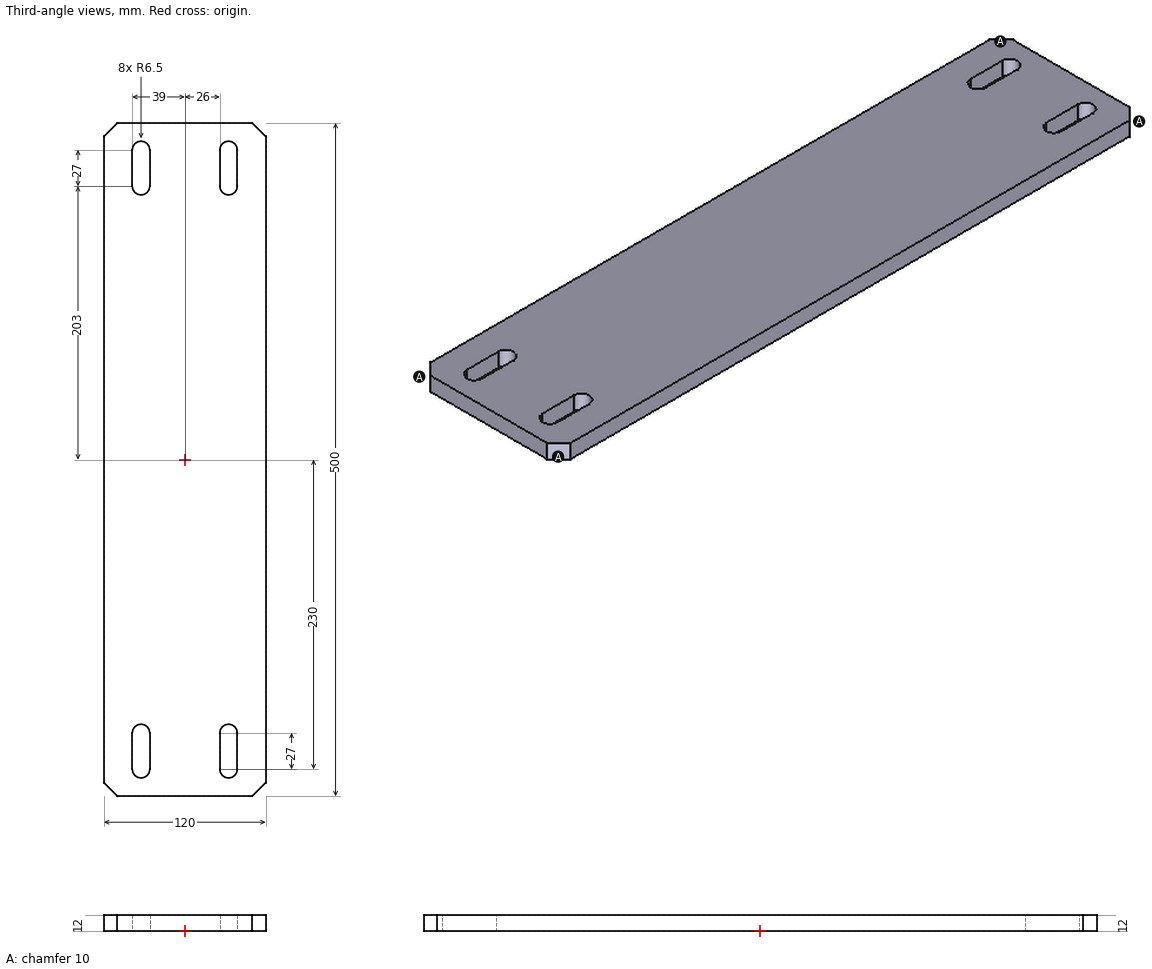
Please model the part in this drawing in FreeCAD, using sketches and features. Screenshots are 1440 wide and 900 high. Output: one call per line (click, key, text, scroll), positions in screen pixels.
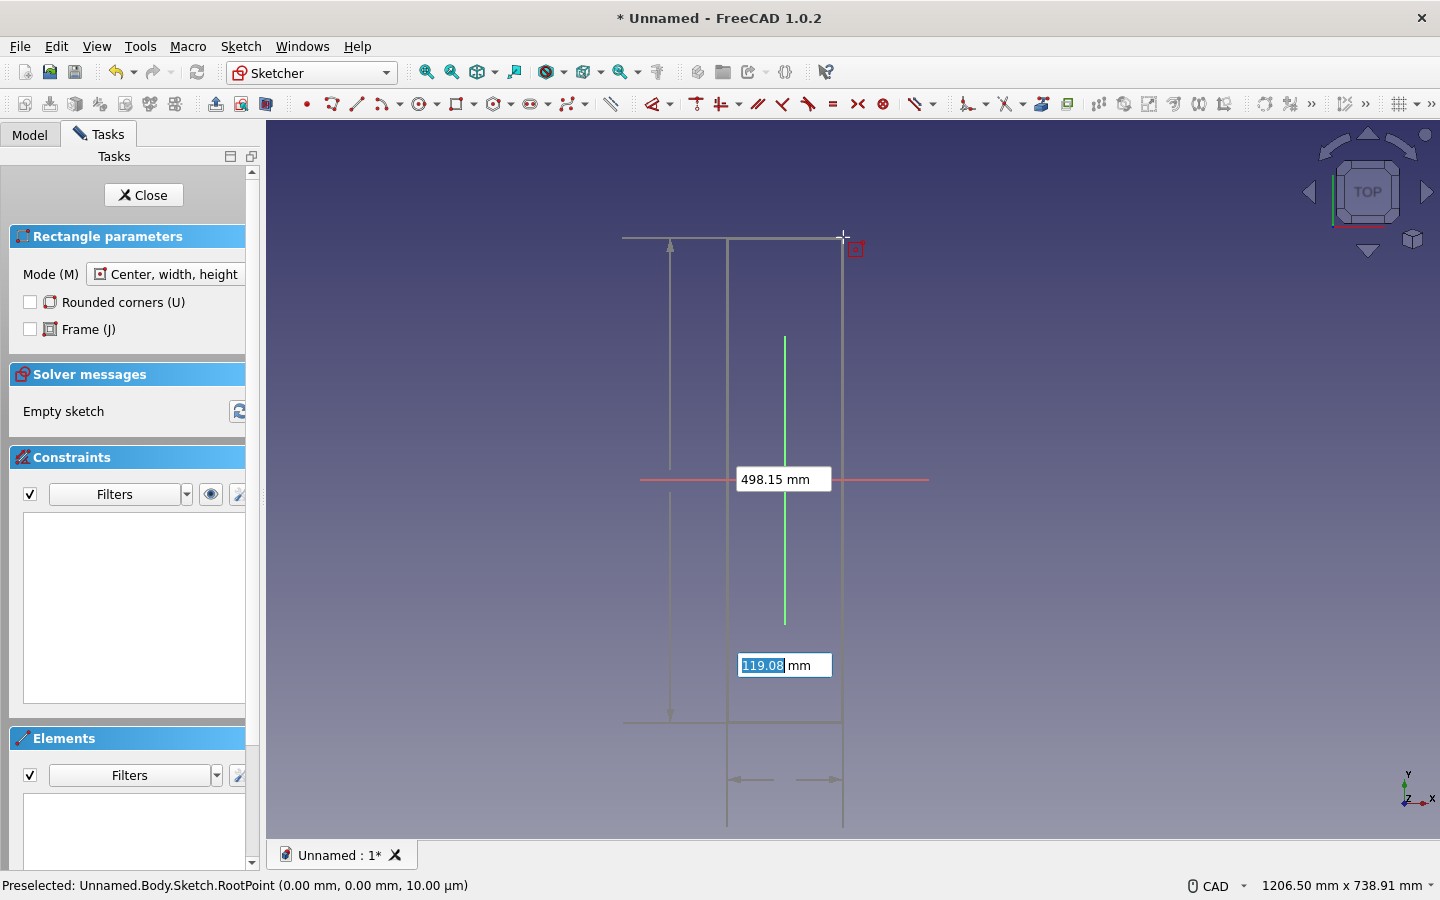
text(120)
key(Tab)
text(500)
key(Return)
key(Escape)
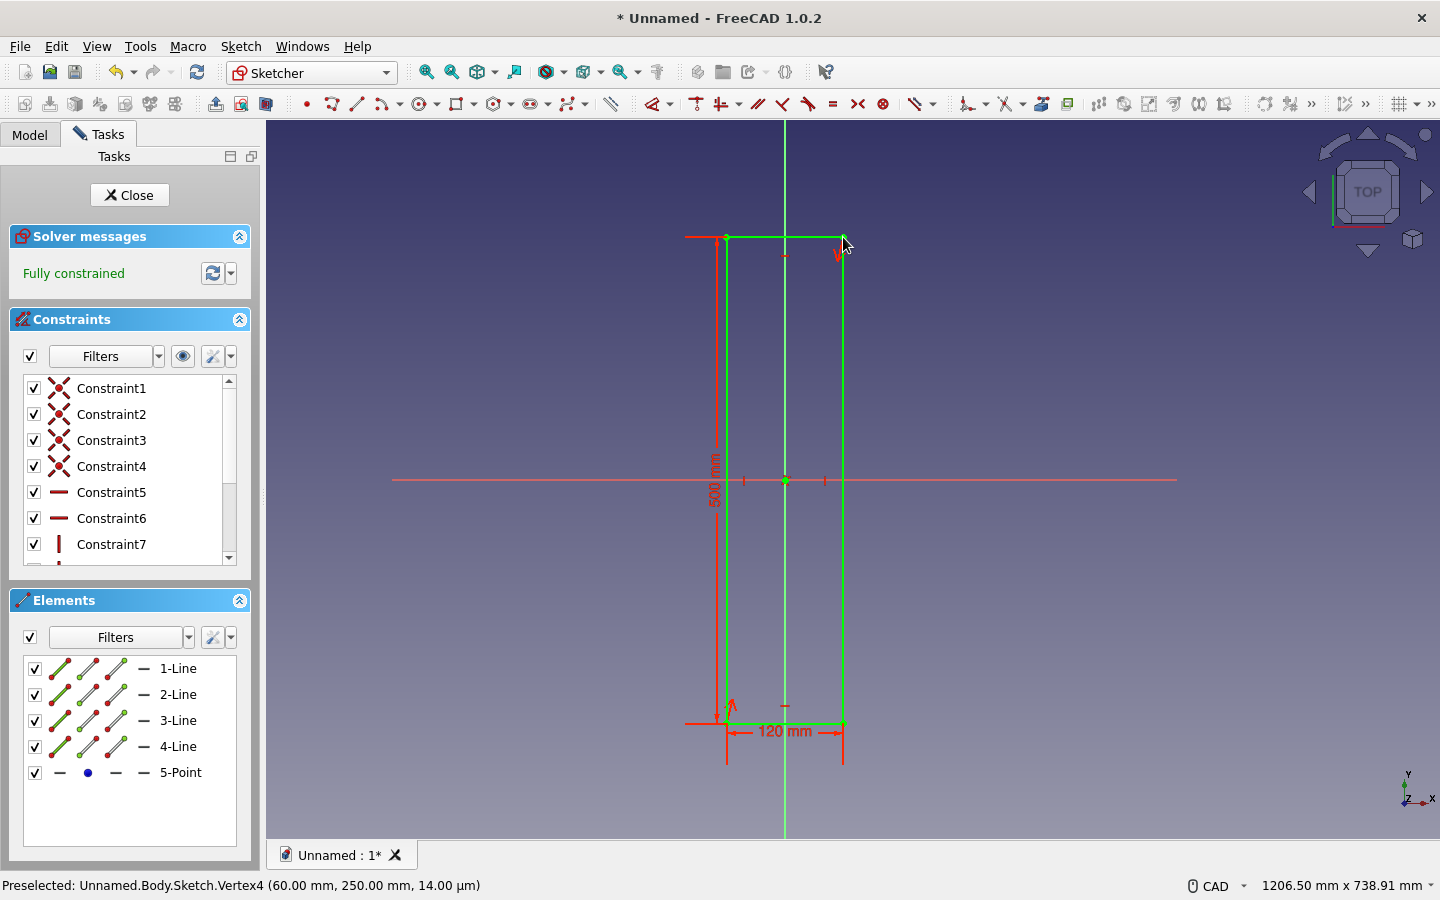
click(130, 195)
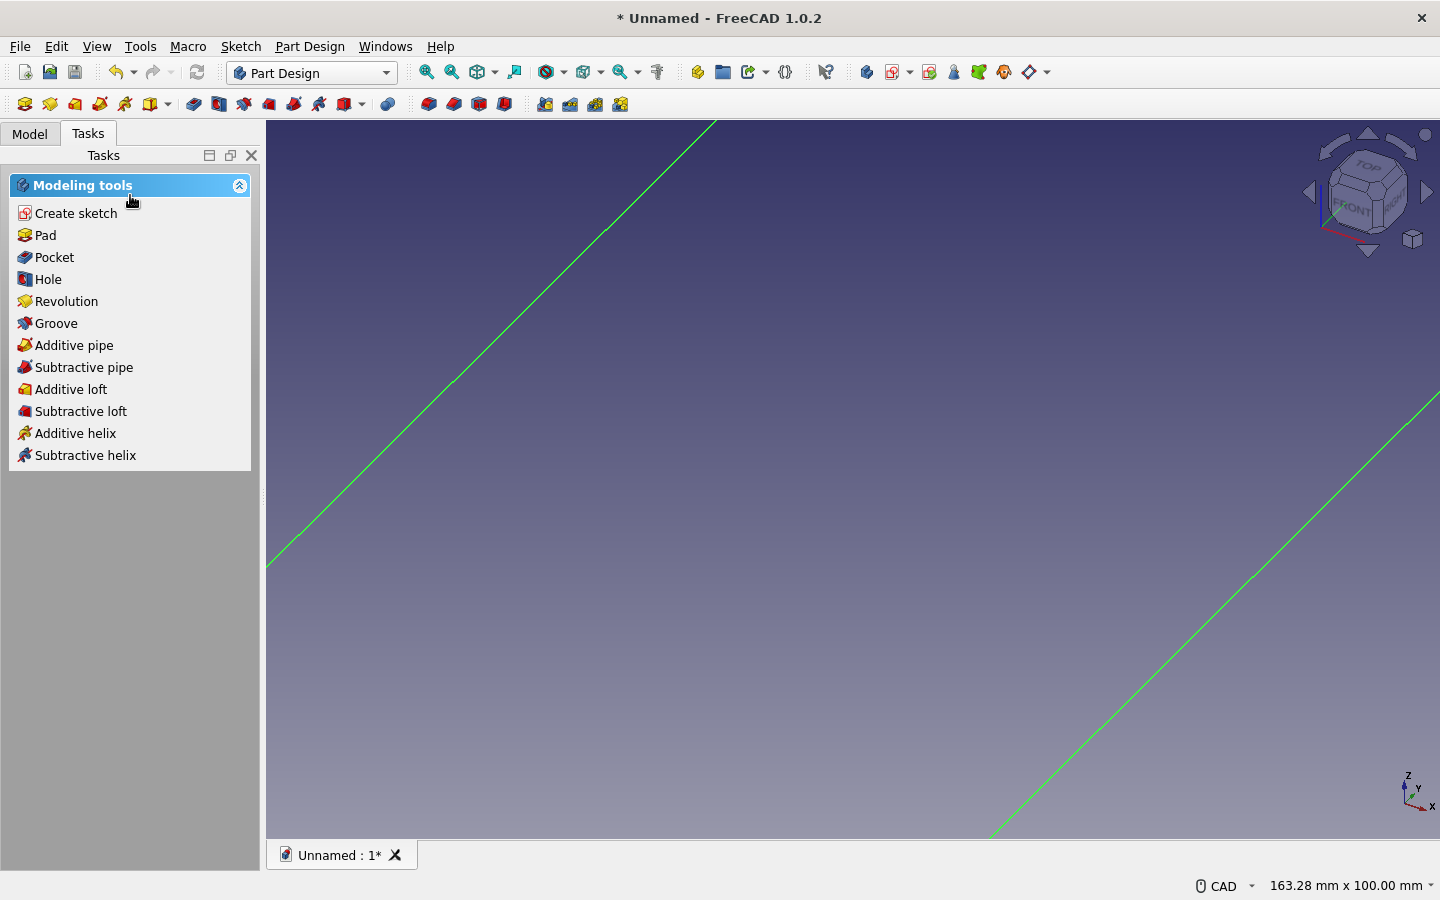
click(25, 104)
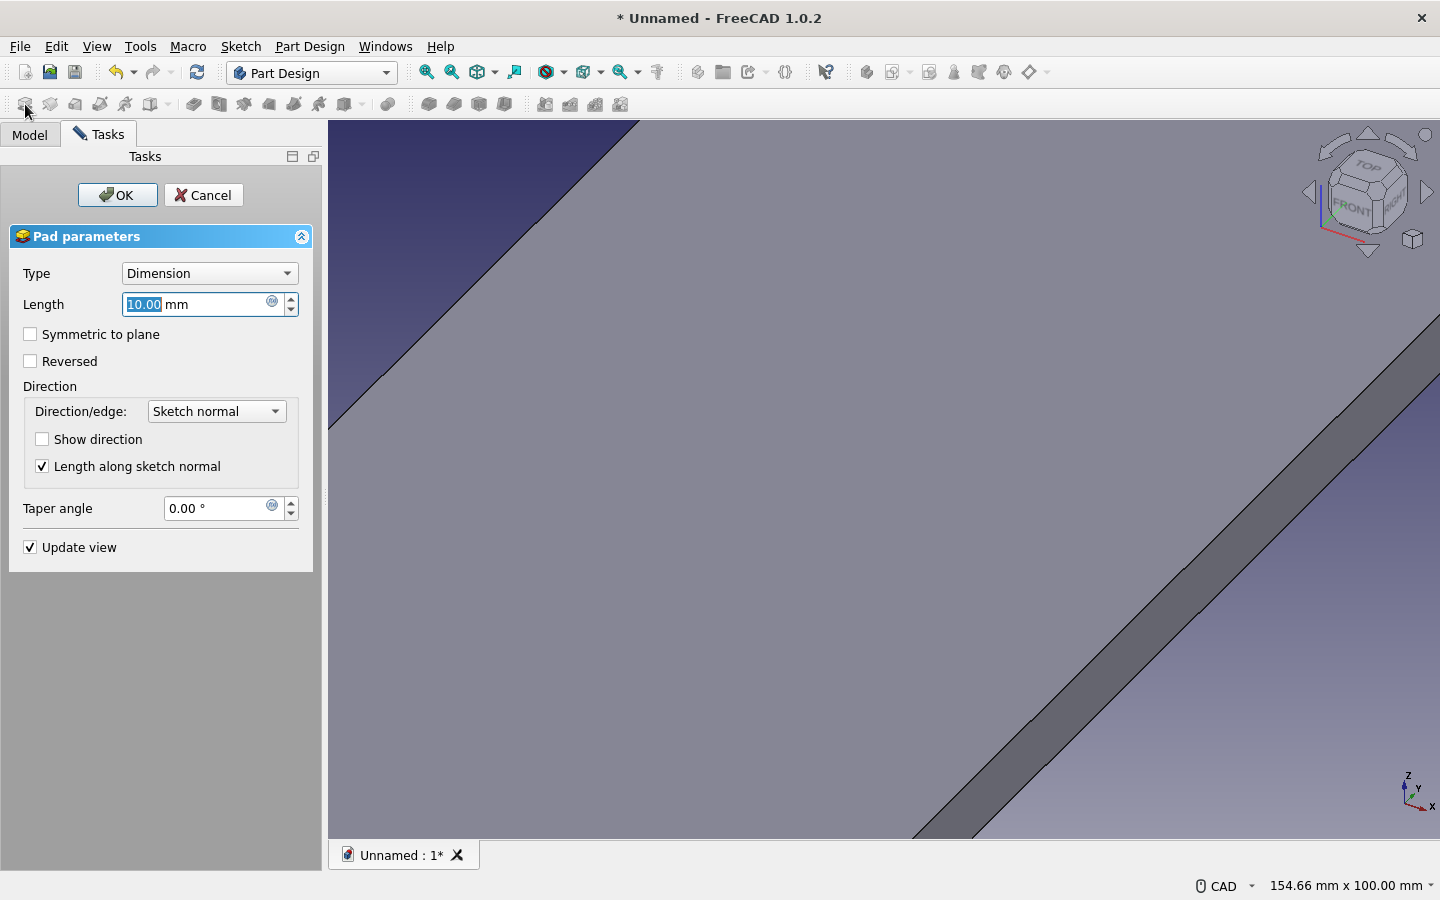
text(12)
key(Tab)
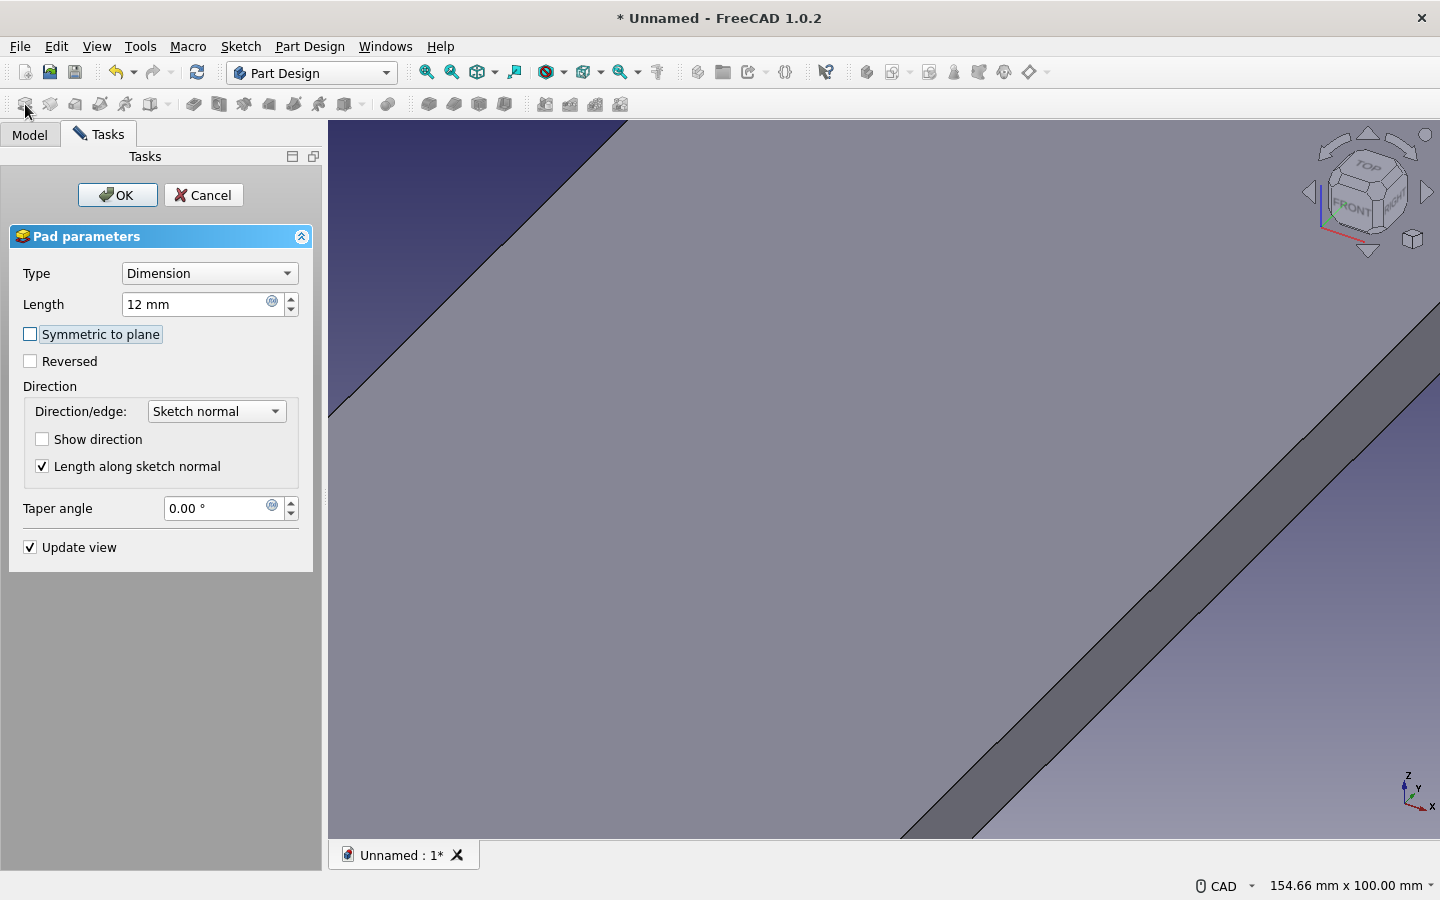
click(118, 195)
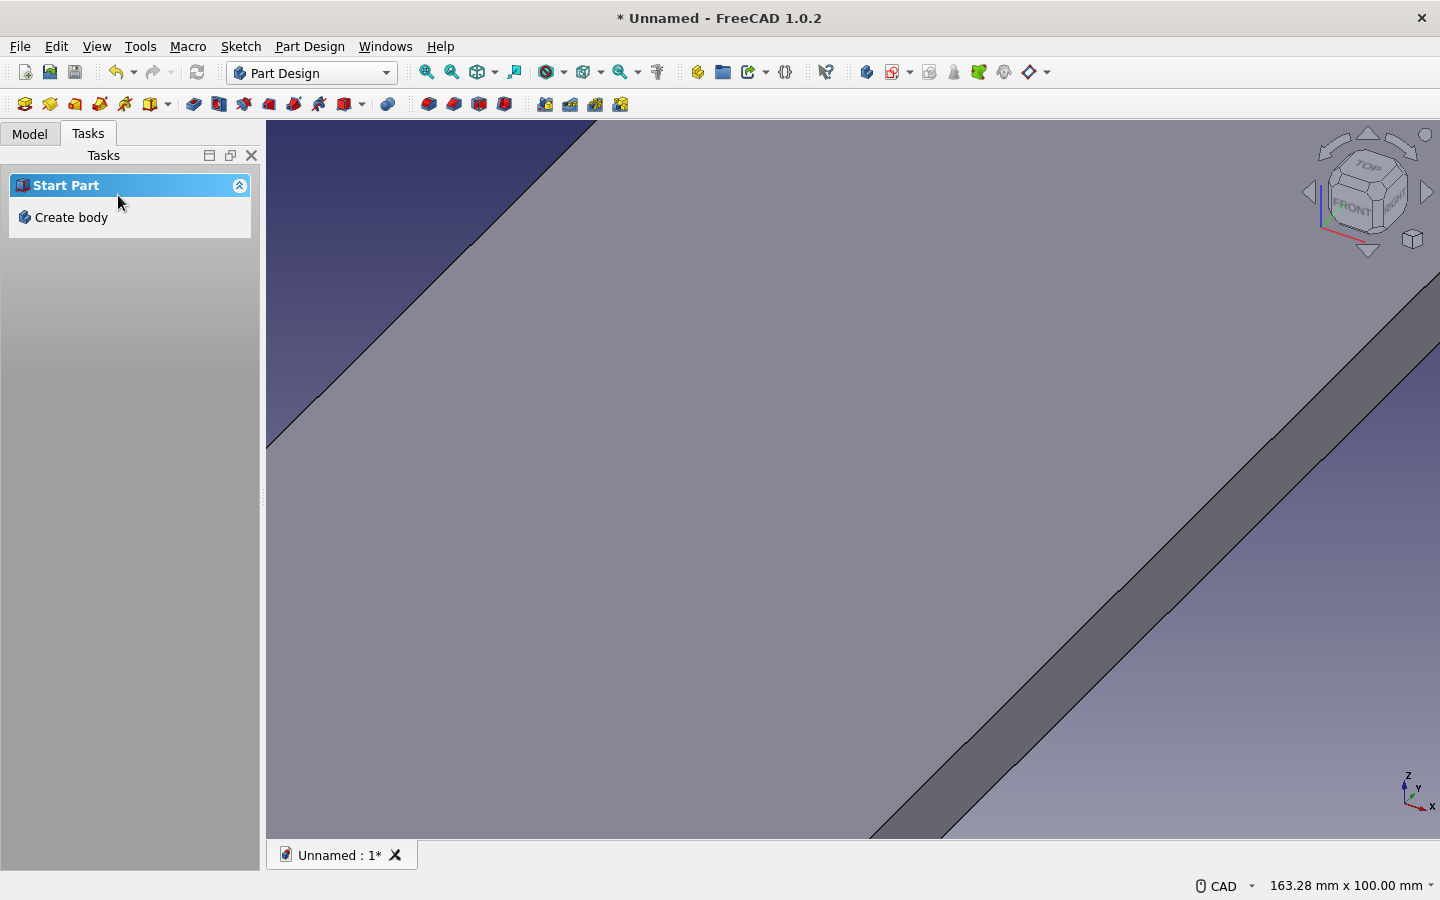
key(v)
key(f)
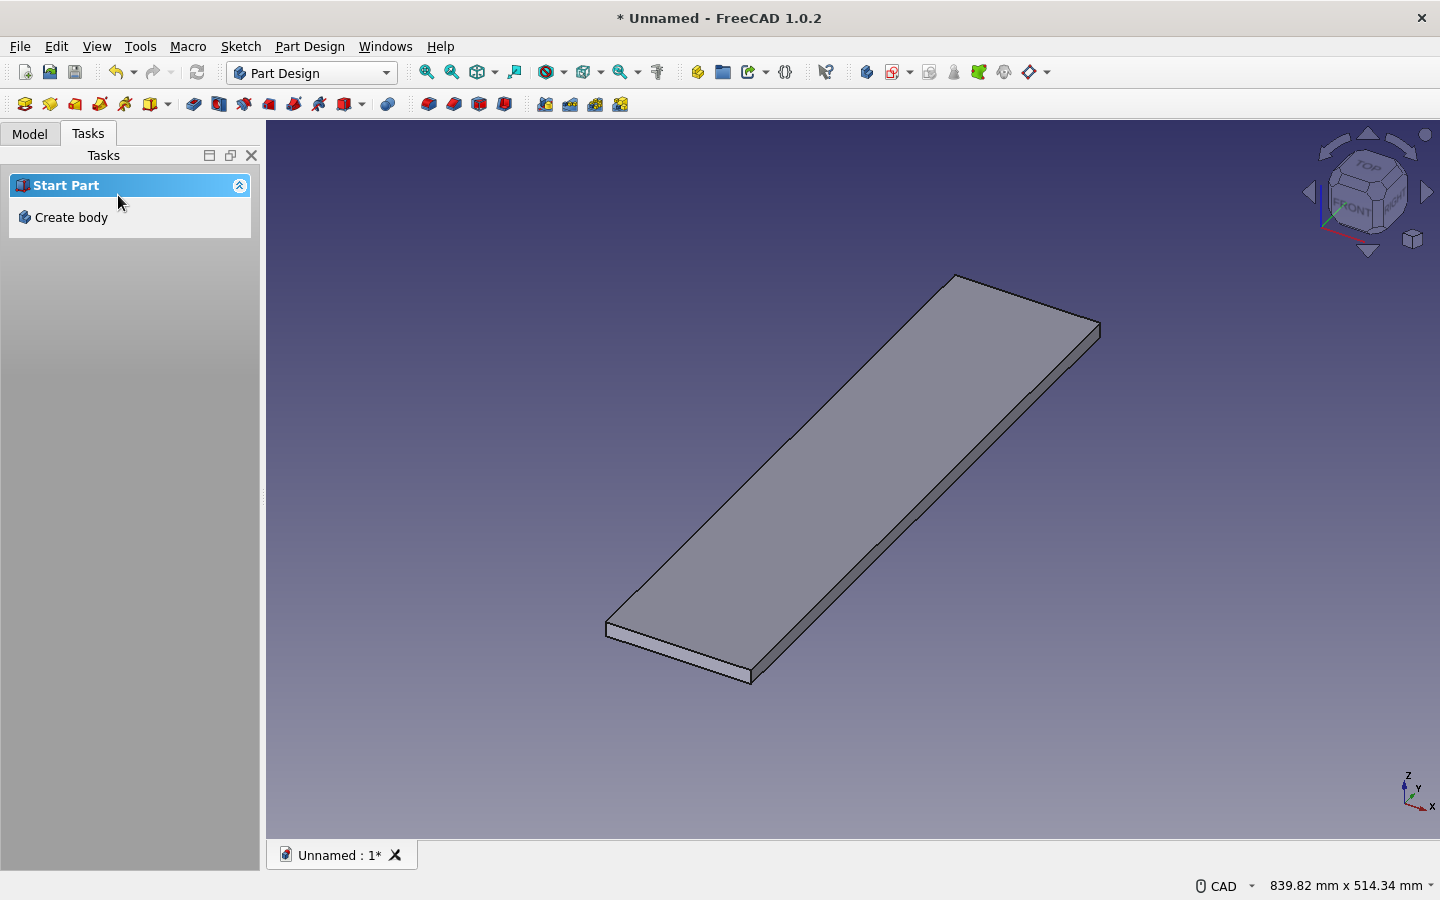
click(953, 372)